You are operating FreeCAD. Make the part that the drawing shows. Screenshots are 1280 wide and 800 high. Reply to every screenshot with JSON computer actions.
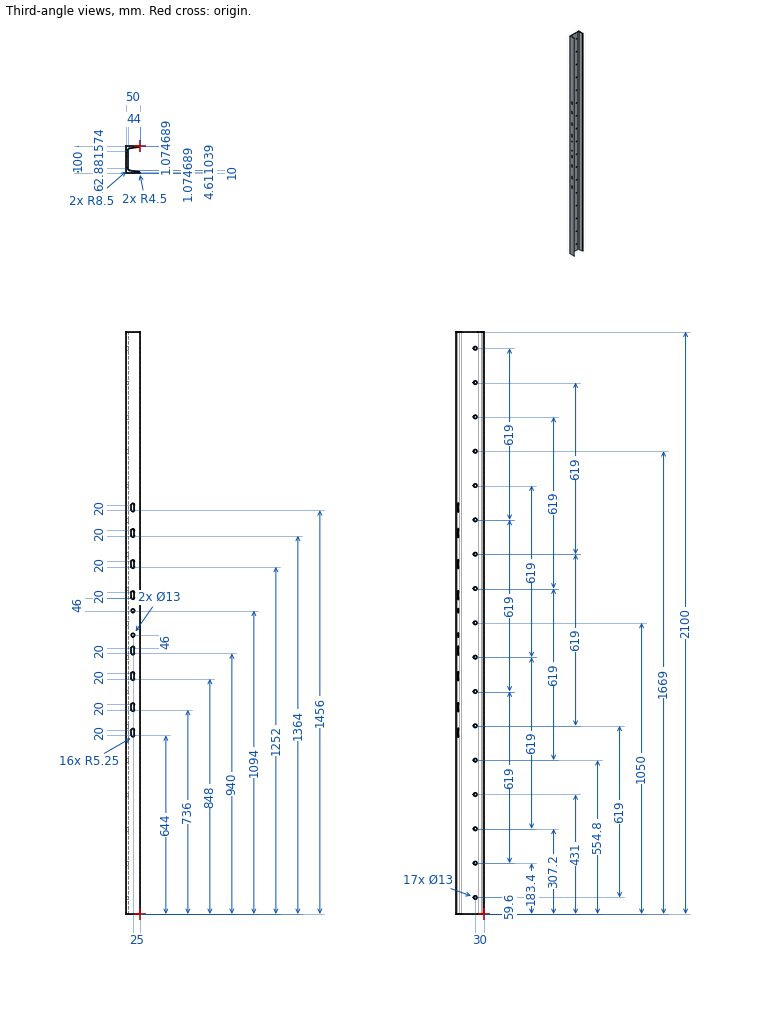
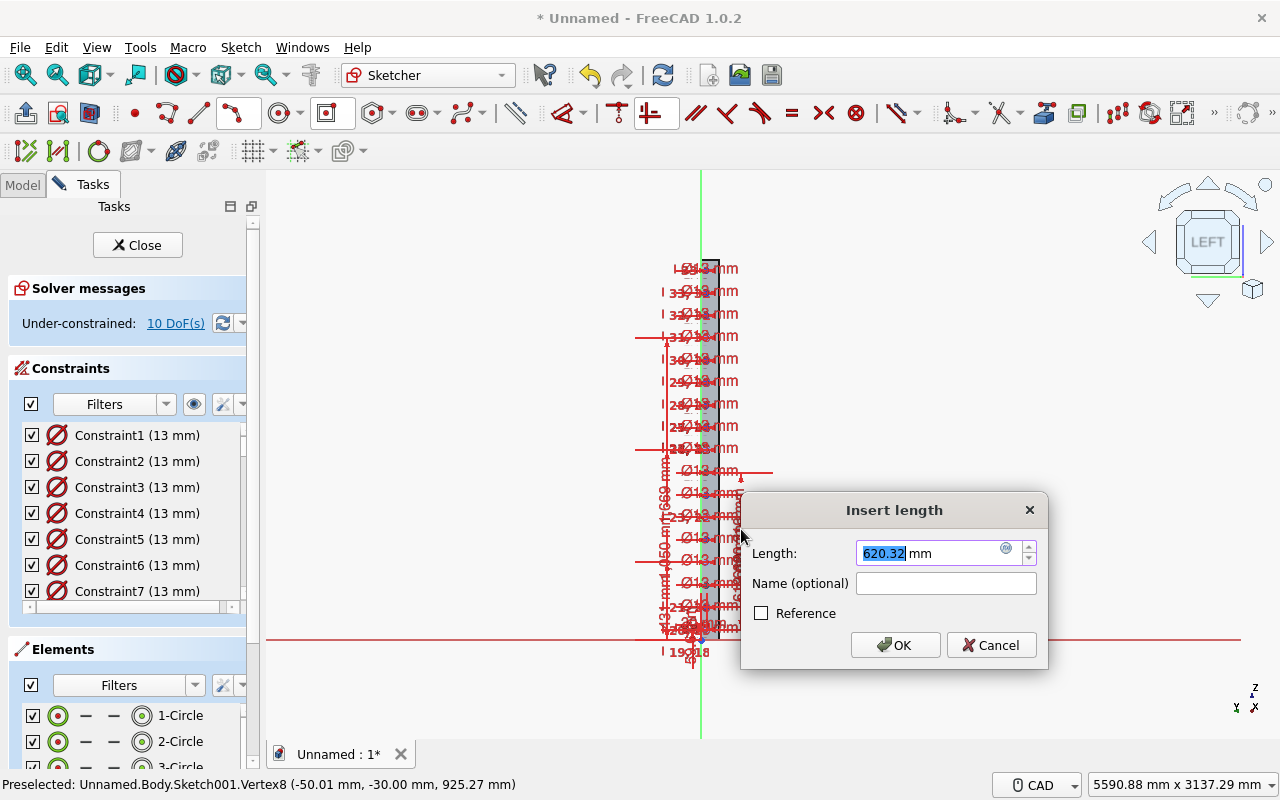
{"action": "type", "text": "619"}
{"action": "key", "text": "Return"}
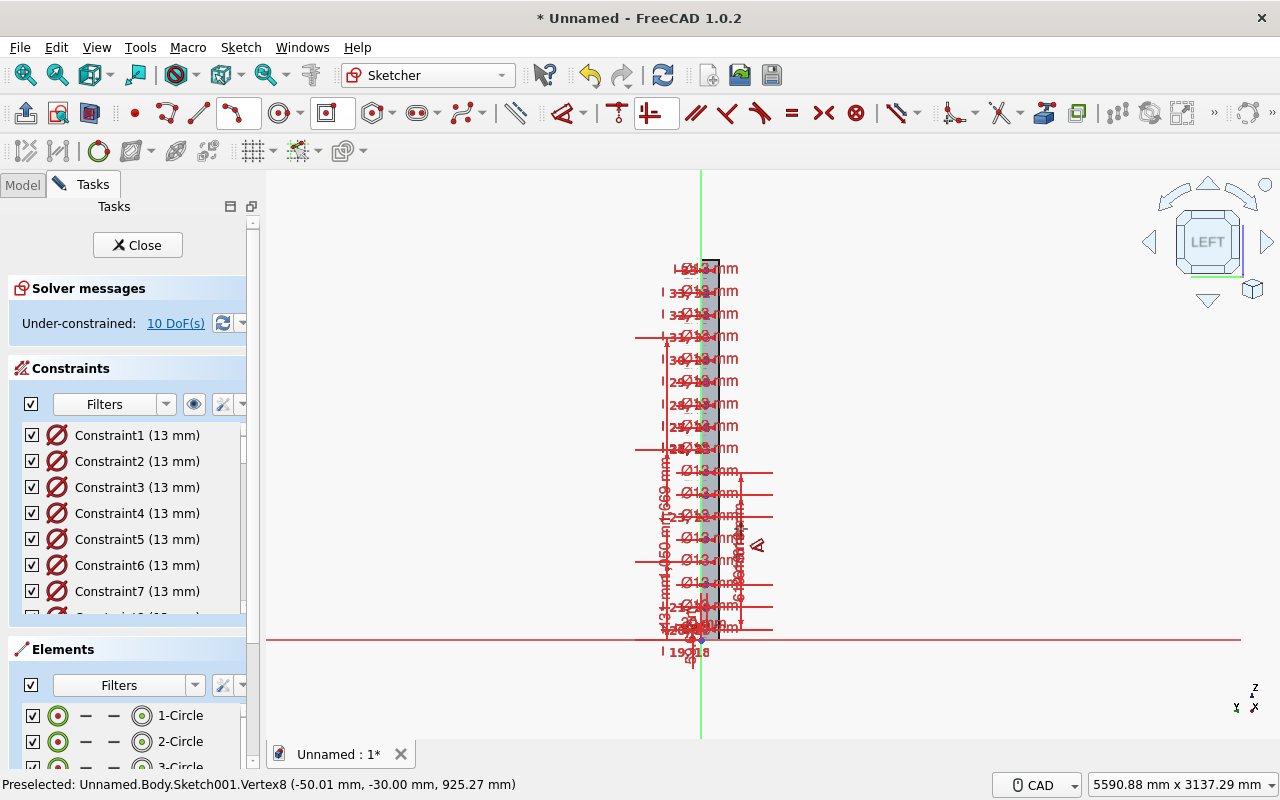
{"action": "left_click", "coordinate": [707, 540]}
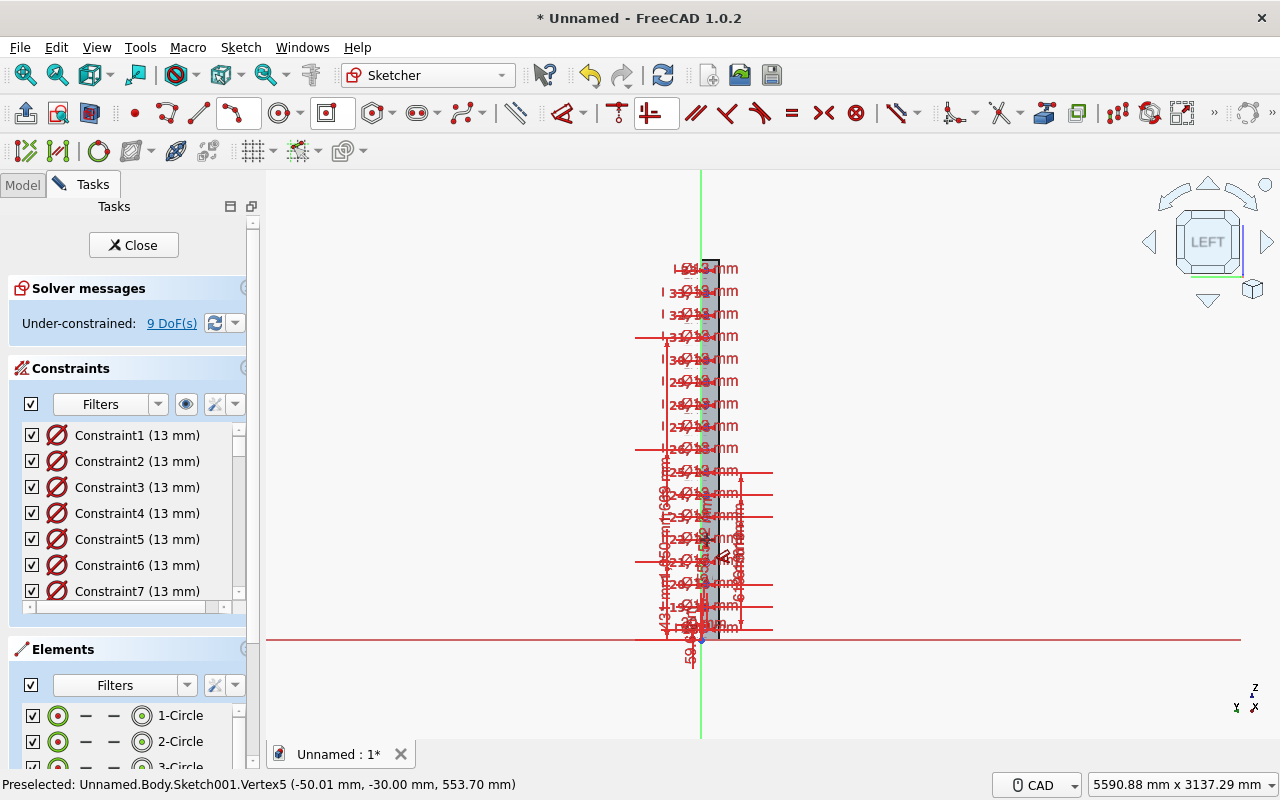
{"action": "left_click", "coordinate": [707, 428]}
{"action": "left_click", "coordinate": [741, 484]}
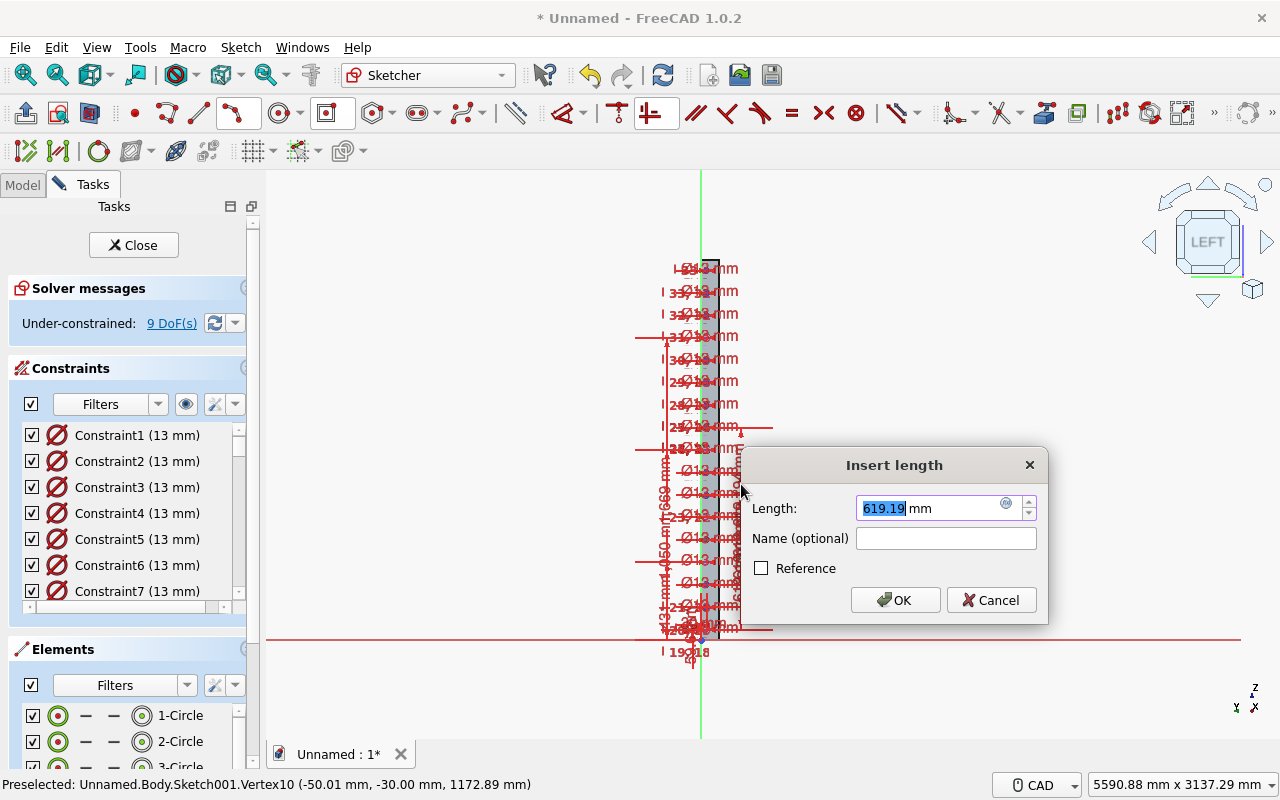
{"action": "type", "text": "619"}
{"action": "key", "text": "Return"}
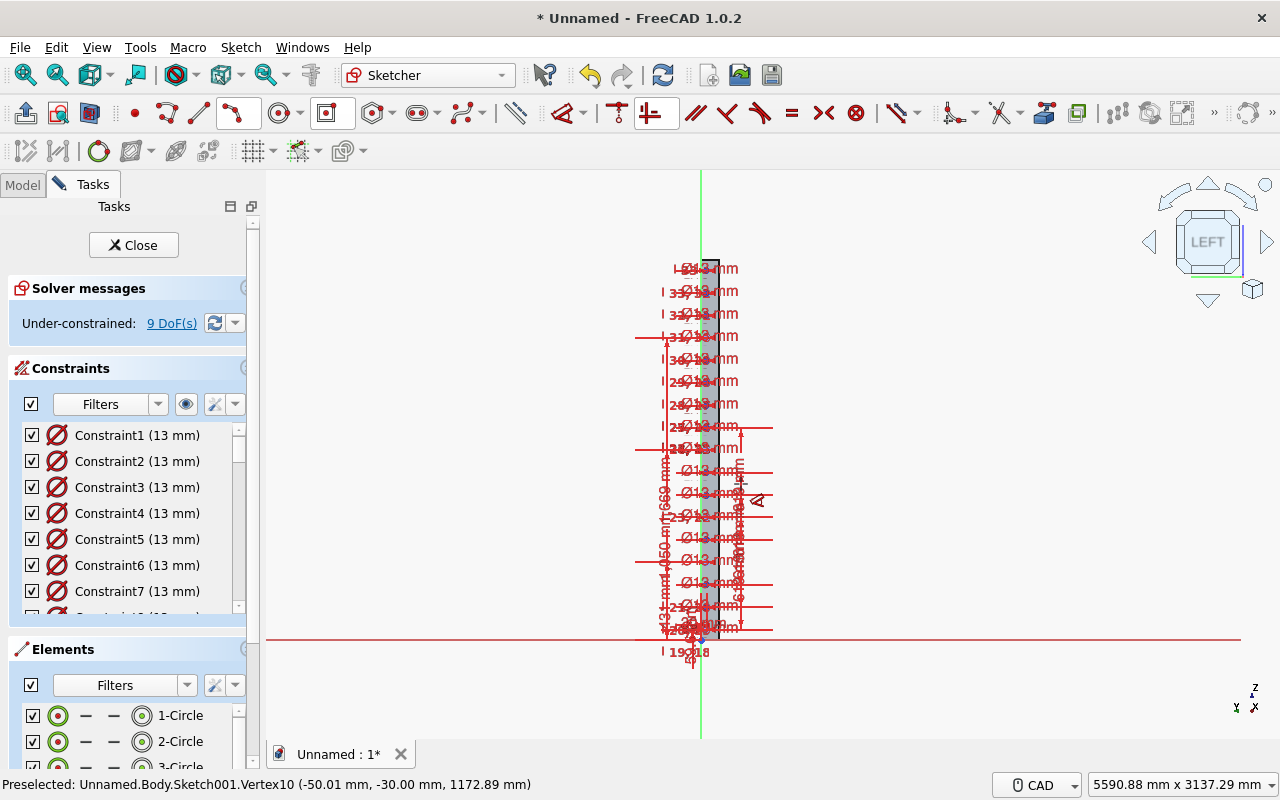
{"action": "left_click", "coordinate": [707, 517]}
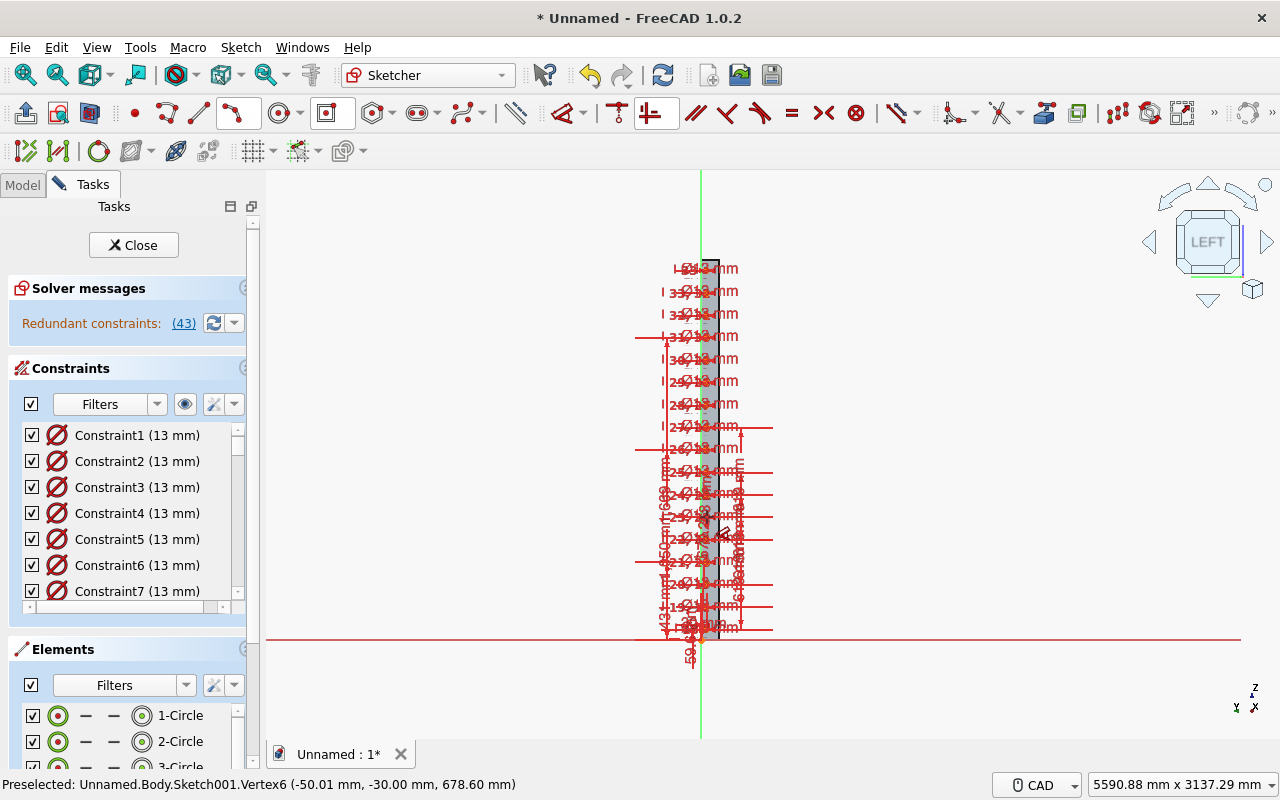
{"action": "left_click", "coordinate": [707, 406]}
{"action": "left_click", "coordinate": [741, 461]}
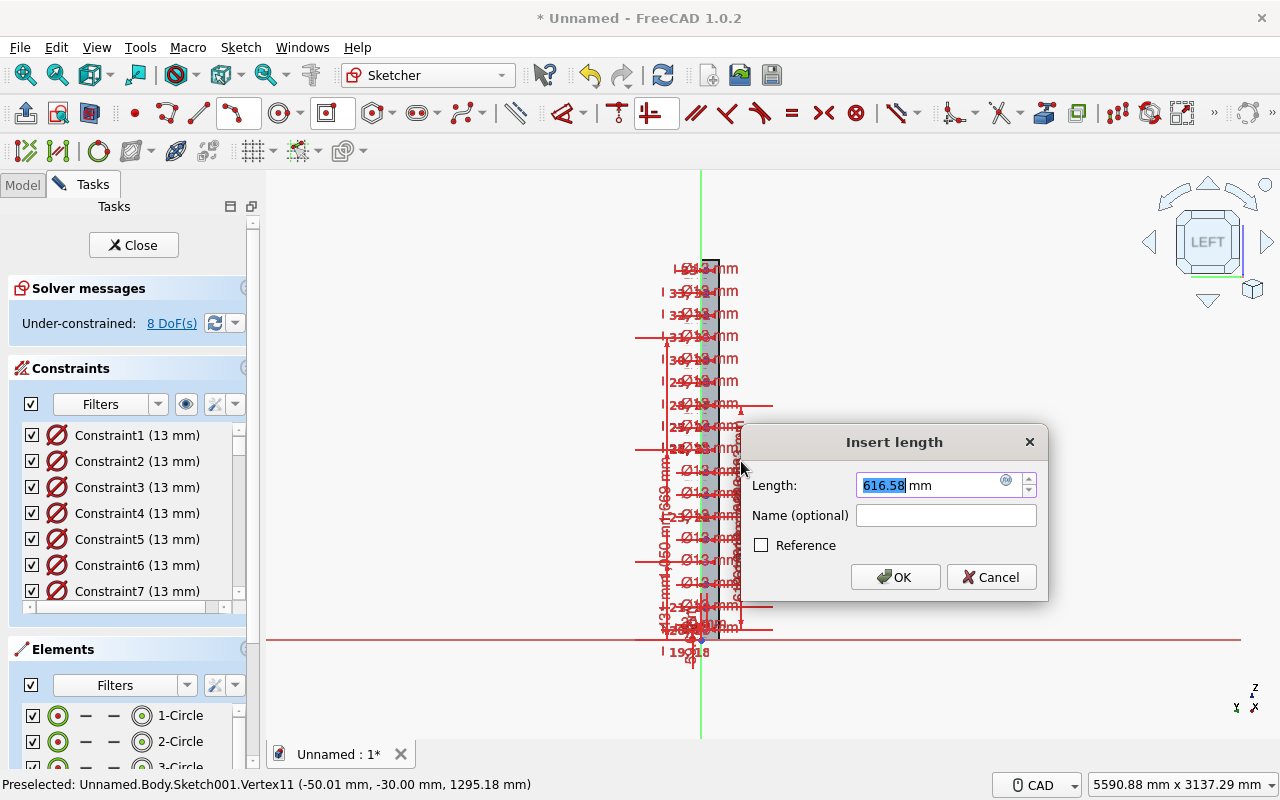
{"action": "type", "text": "619"}
{"action": "key", "text": "Return"}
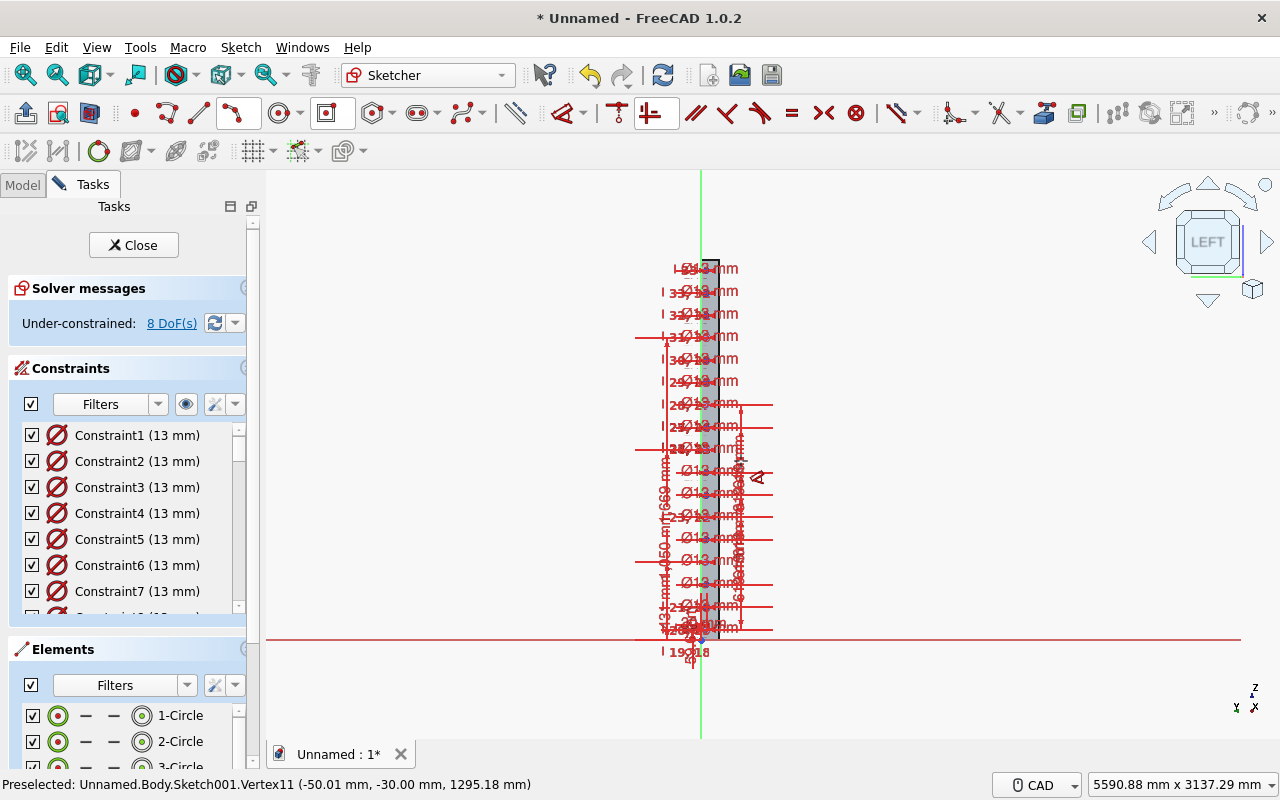
{"action": "left_click", "coordinate": [707, 495]}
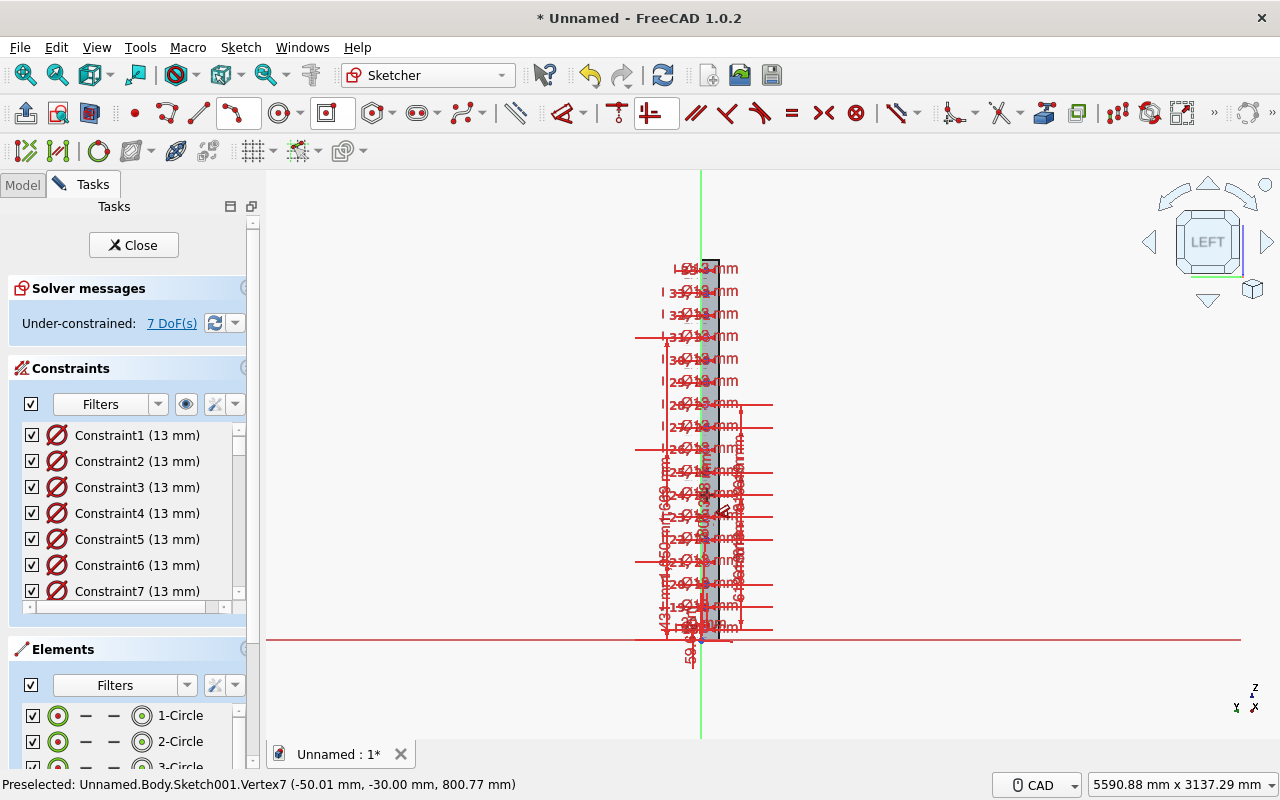
{"action": "left_click", "coordinate": [707, 383]}
{"action": "left_click", "coordinate": [741, 439]}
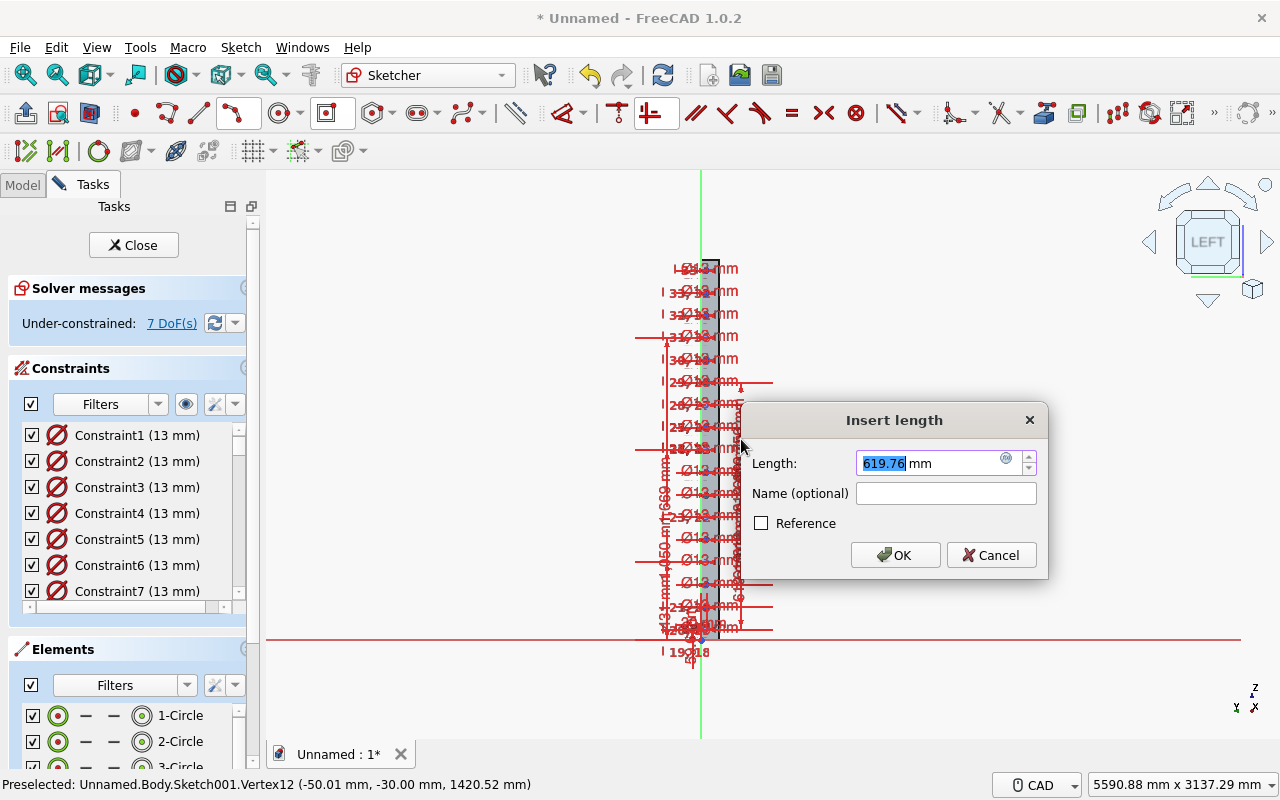
{"action": "type", "text": "619"}
{"action": "key", "text": "Return"}